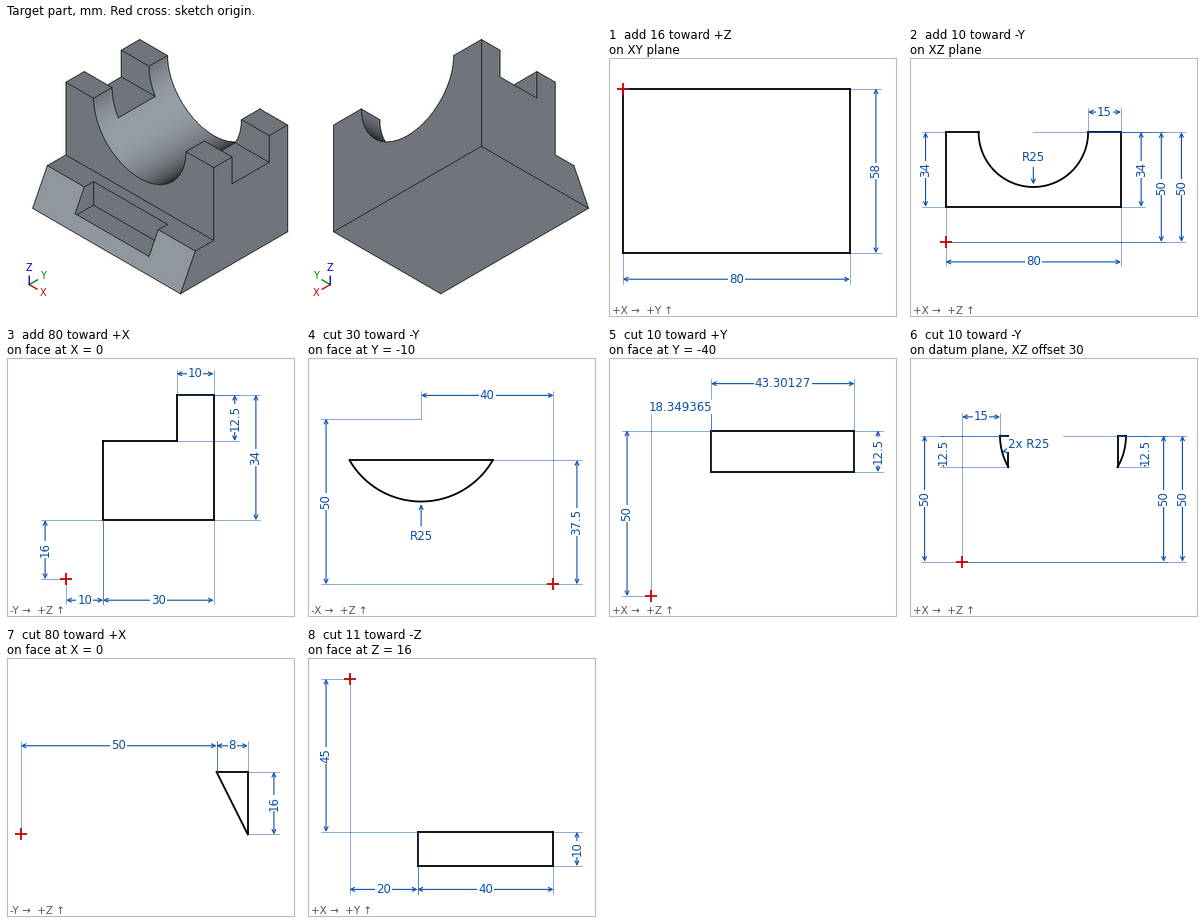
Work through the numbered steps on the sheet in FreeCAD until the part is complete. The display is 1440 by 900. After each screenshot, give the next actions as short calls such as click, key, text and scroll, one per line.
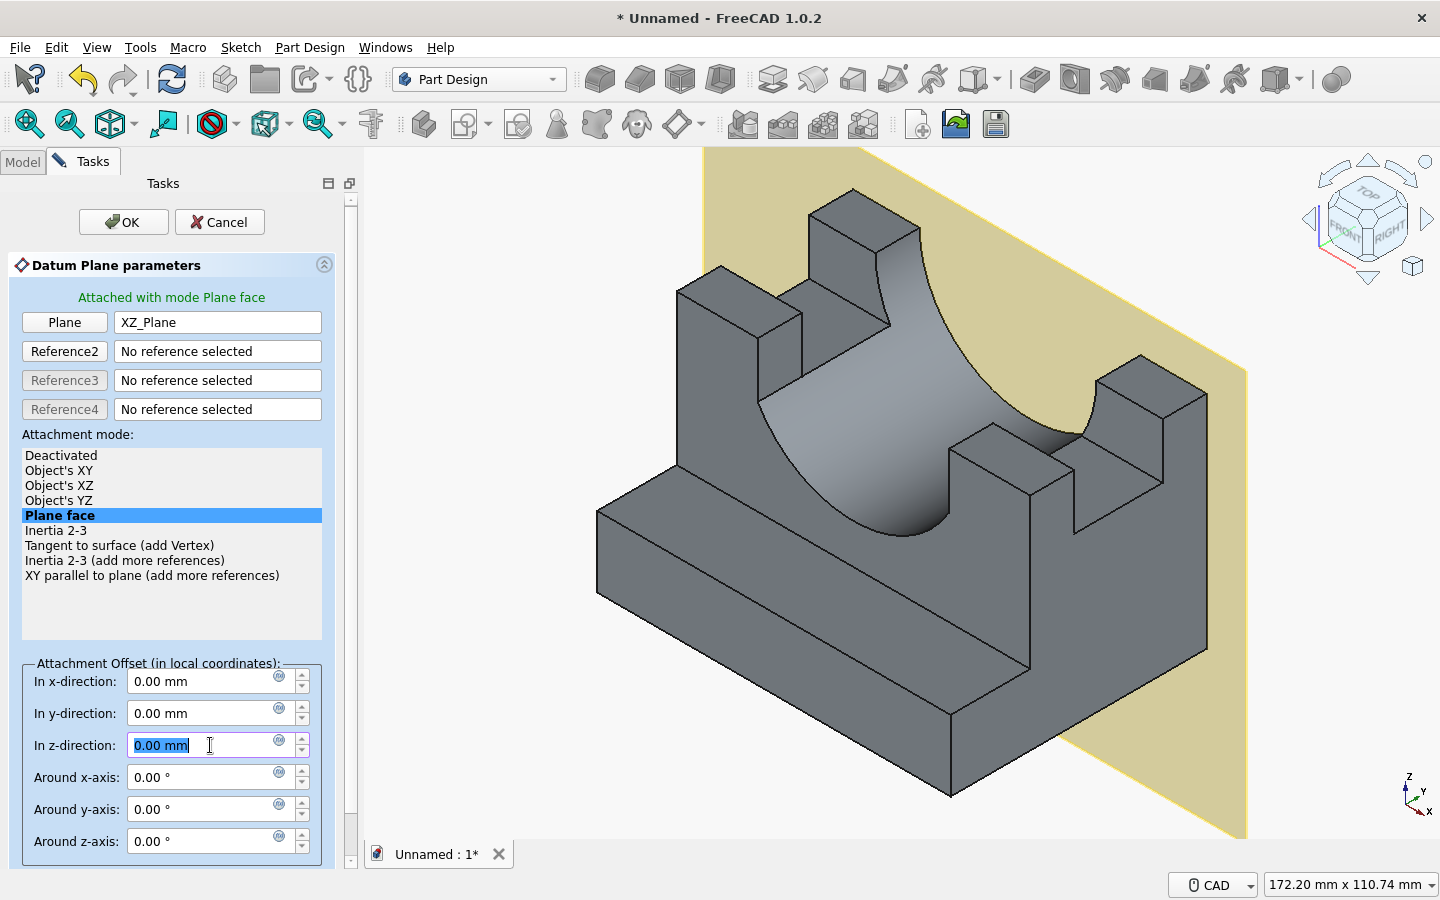
text(30)
key(Tab)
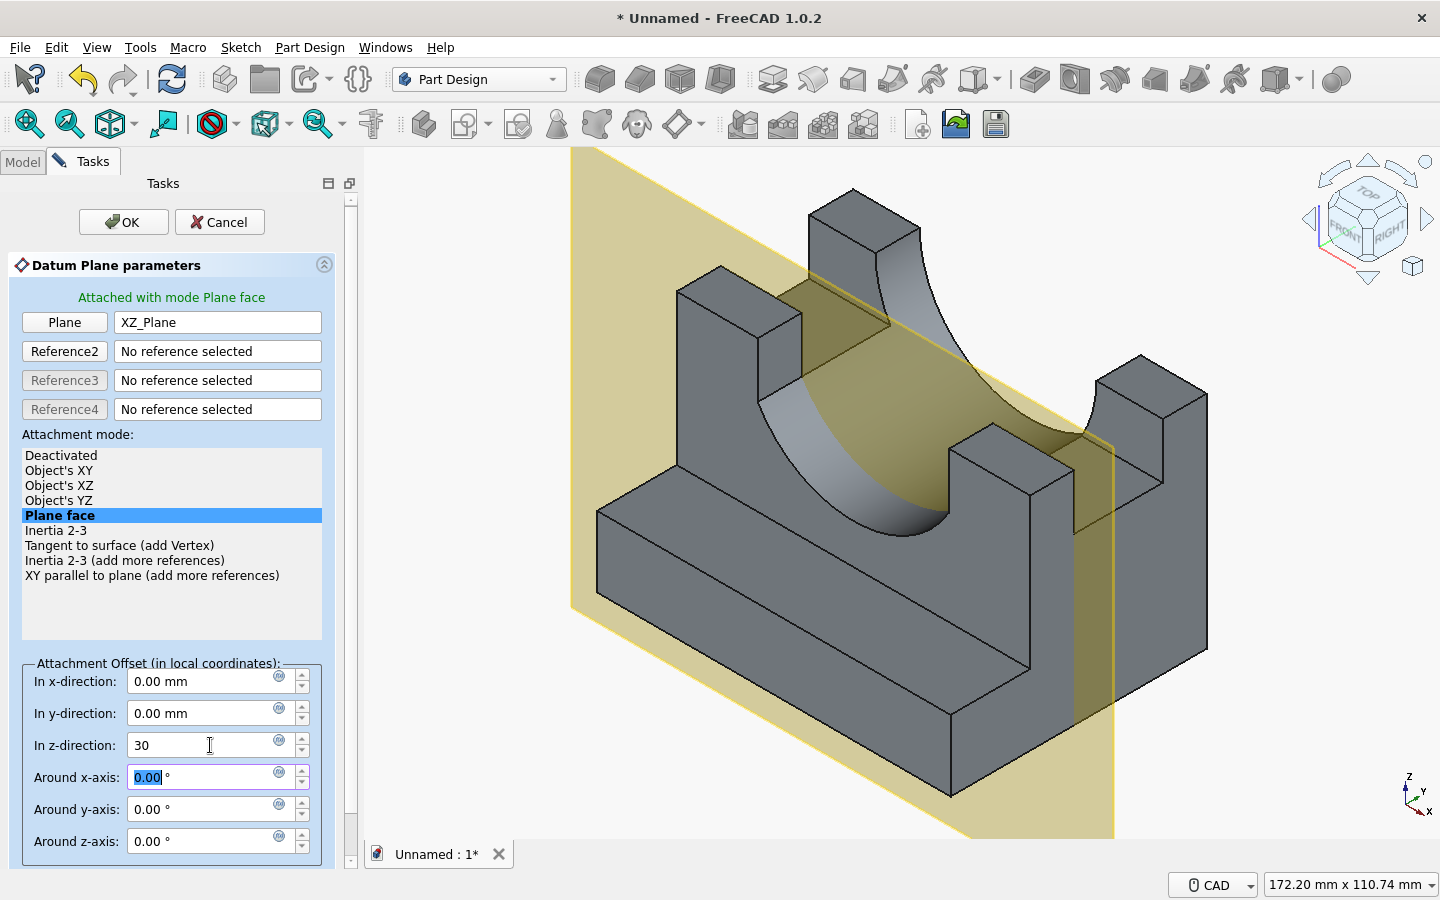
click(124, 222)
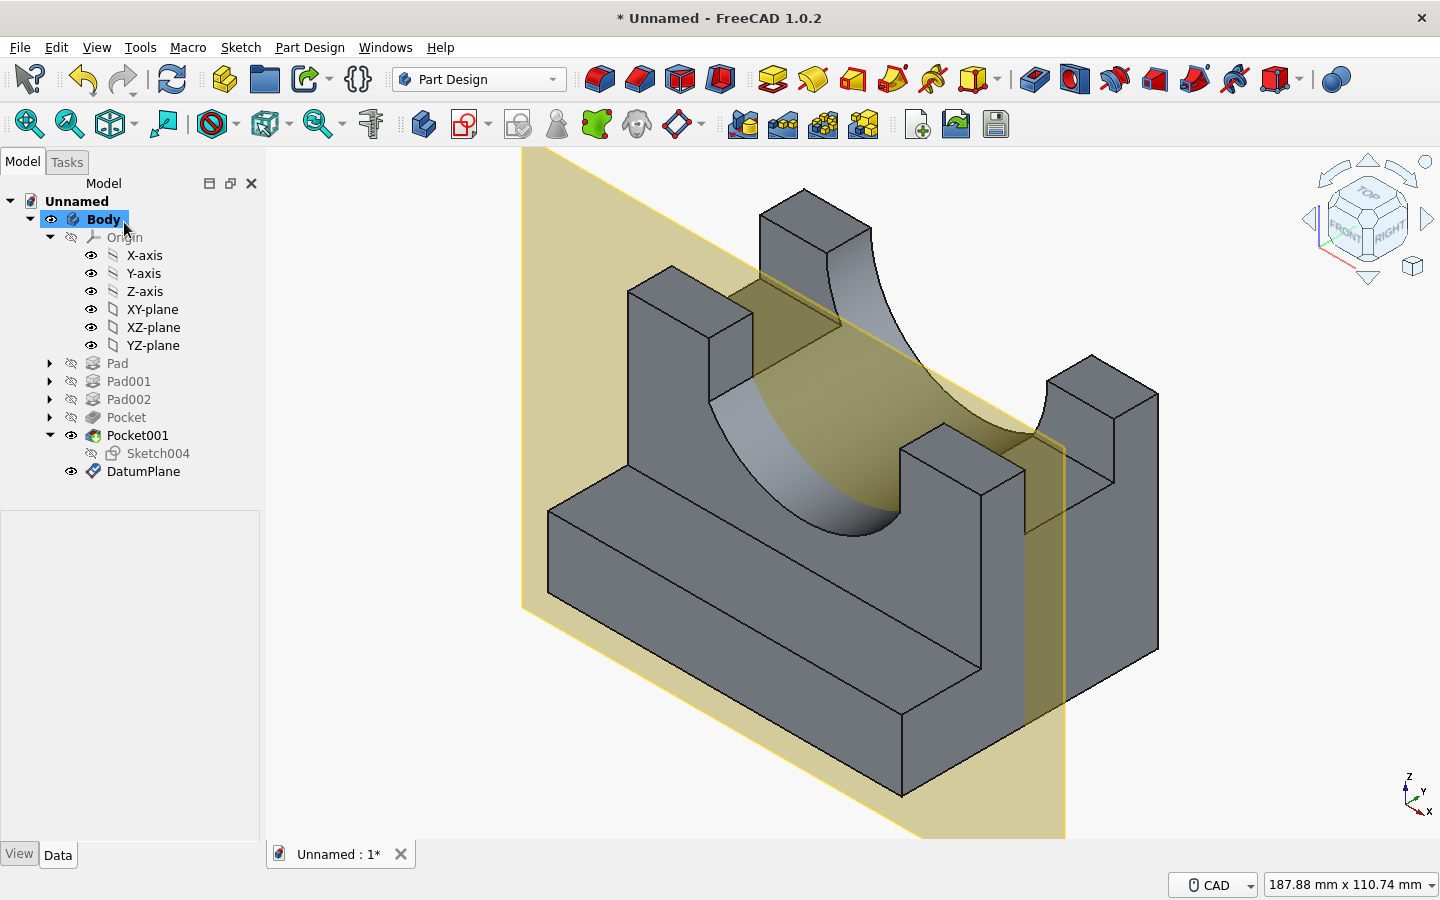
click(116, 471)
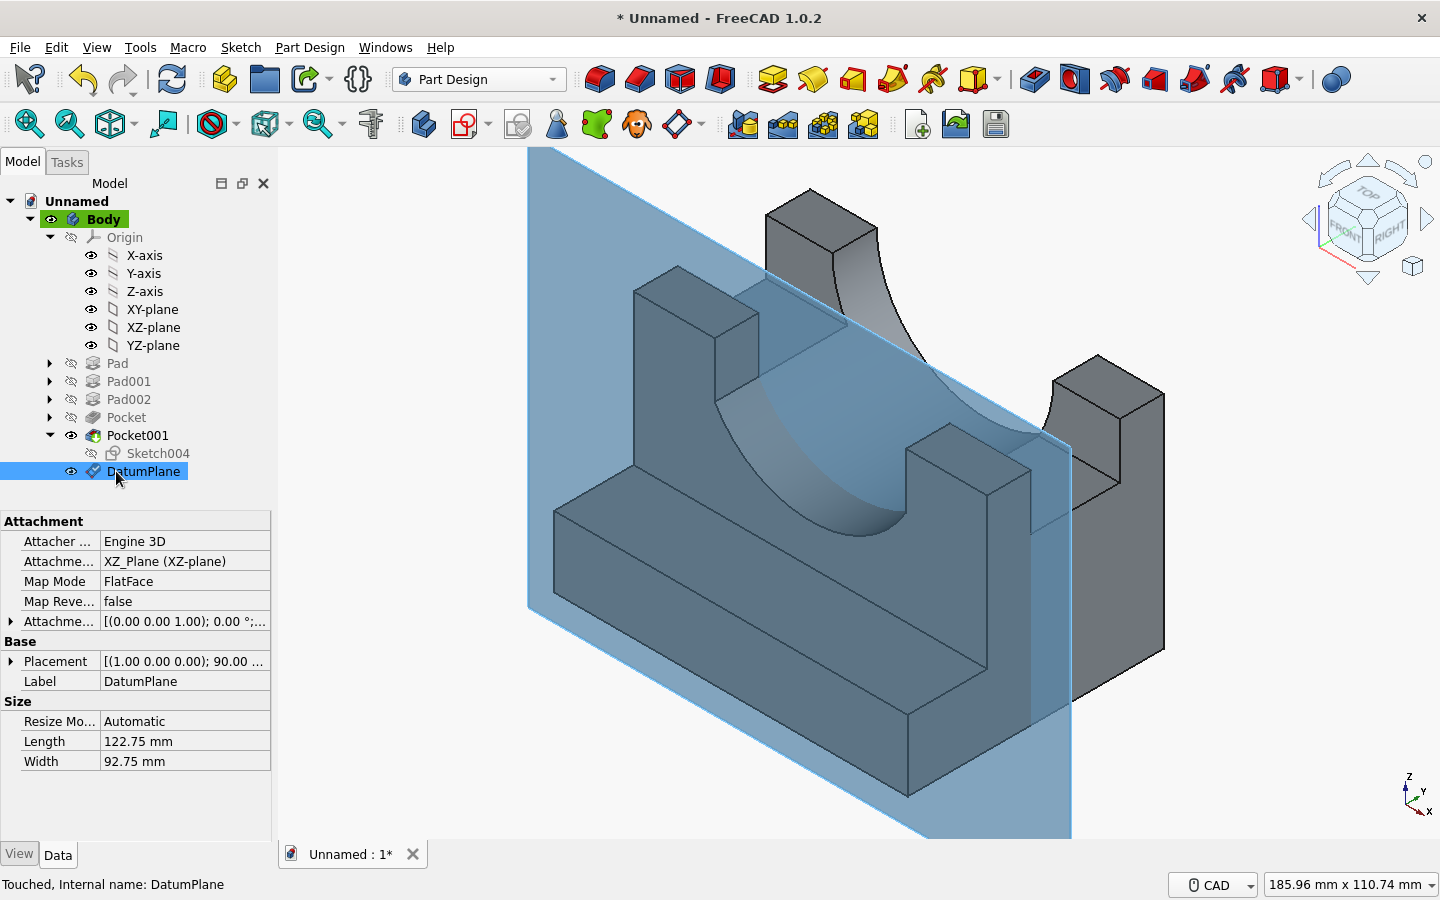
click(464, 124)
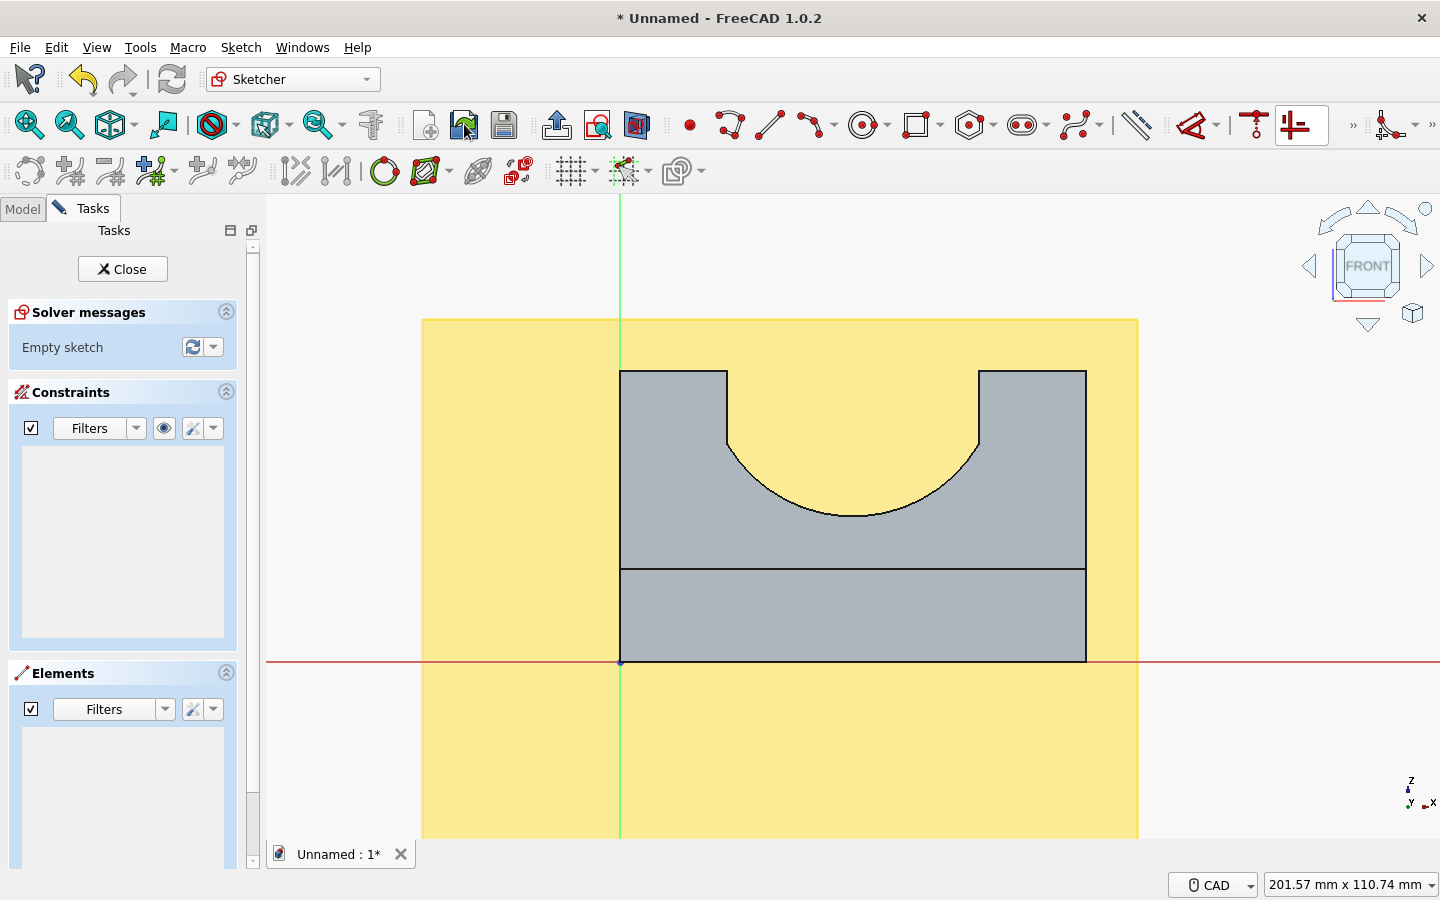
click(638, 126)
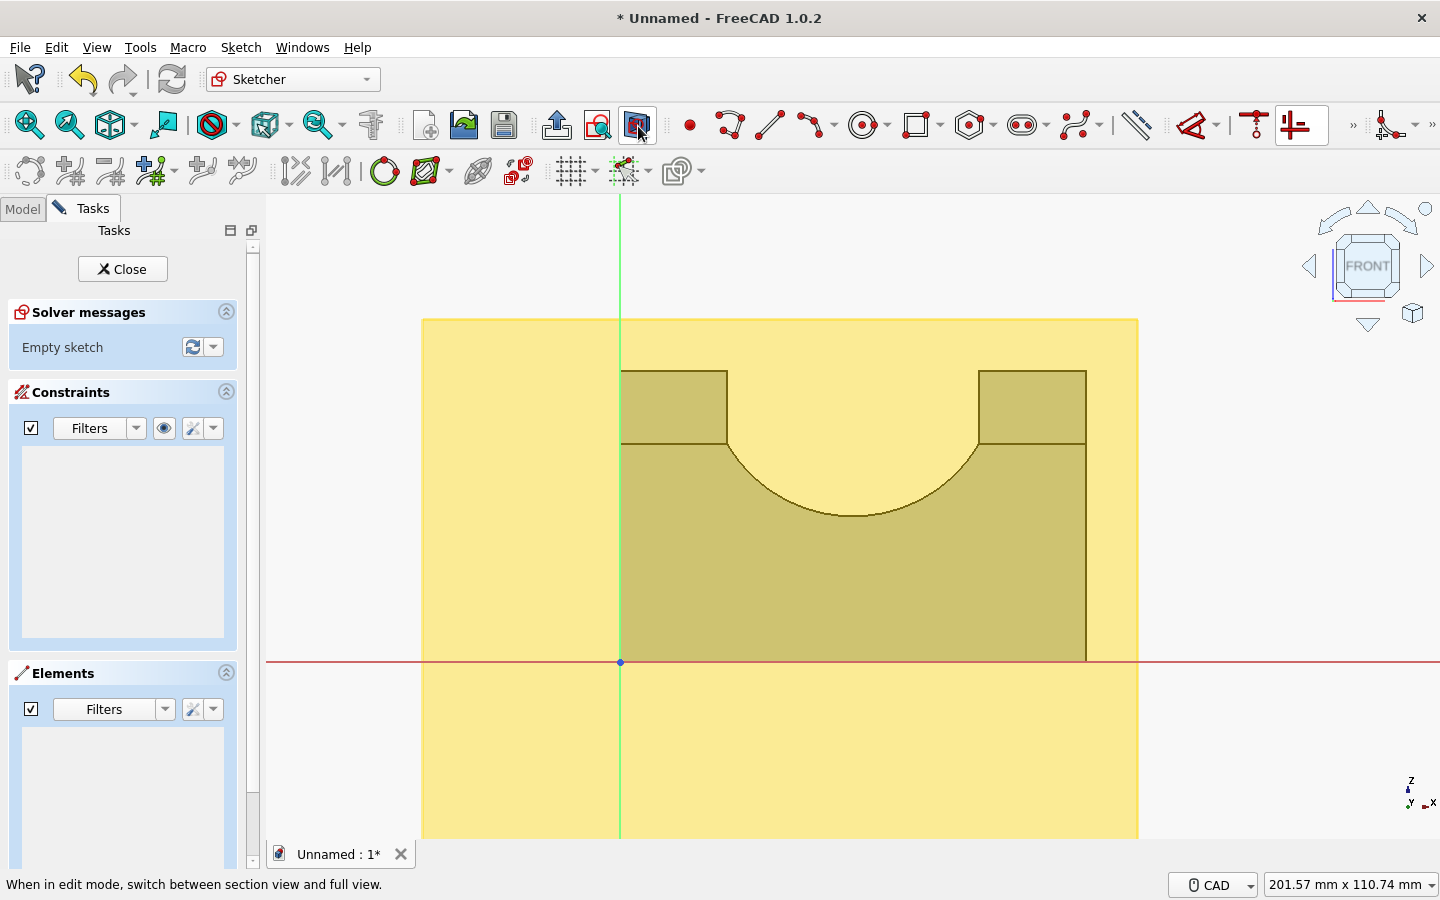
scroll(860, 517, up, 2)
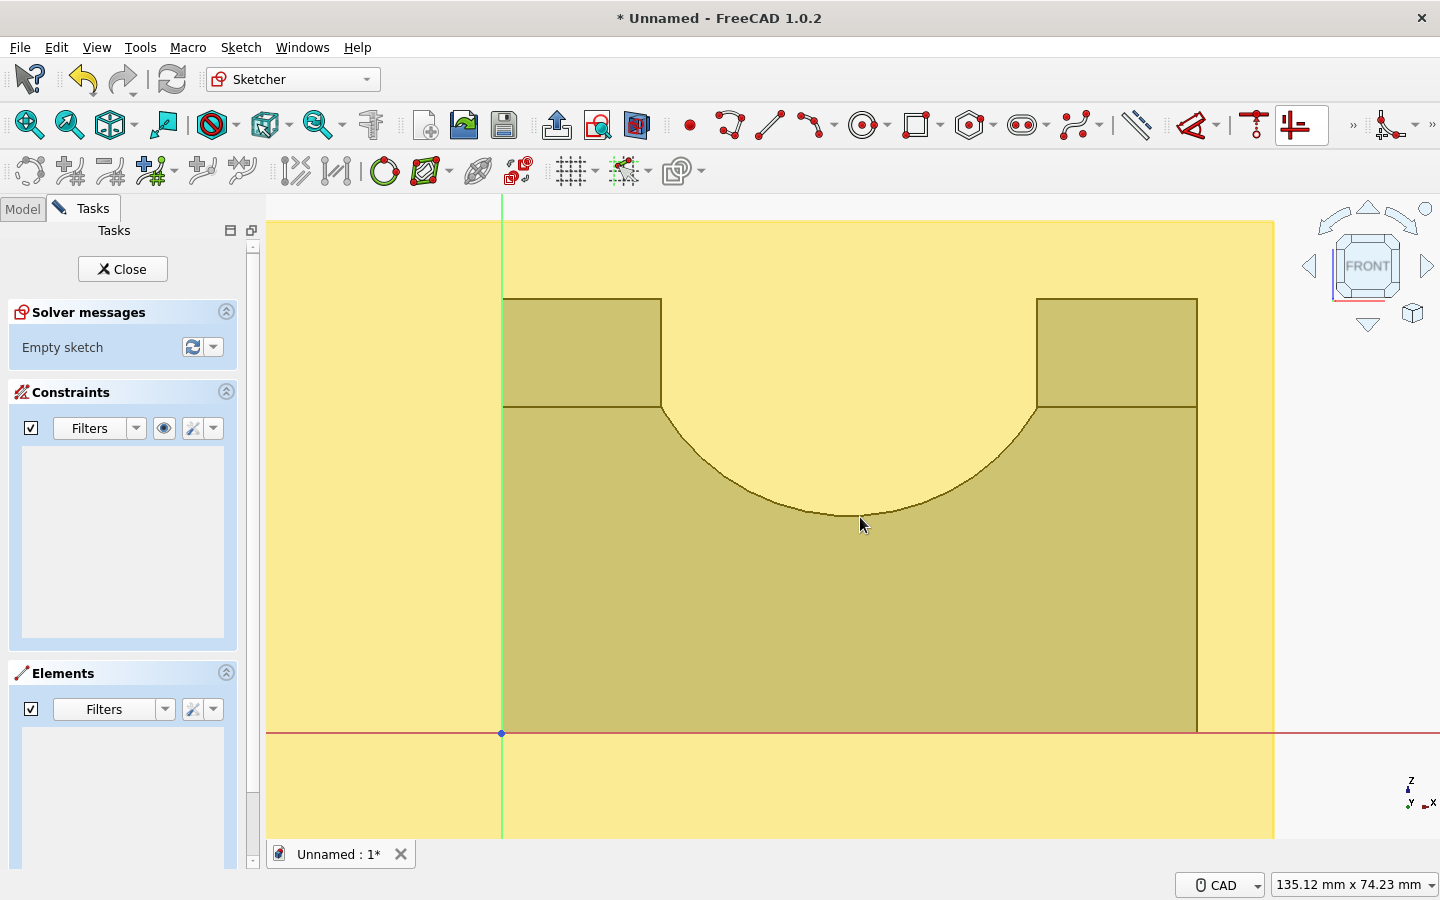
click(730, 126)